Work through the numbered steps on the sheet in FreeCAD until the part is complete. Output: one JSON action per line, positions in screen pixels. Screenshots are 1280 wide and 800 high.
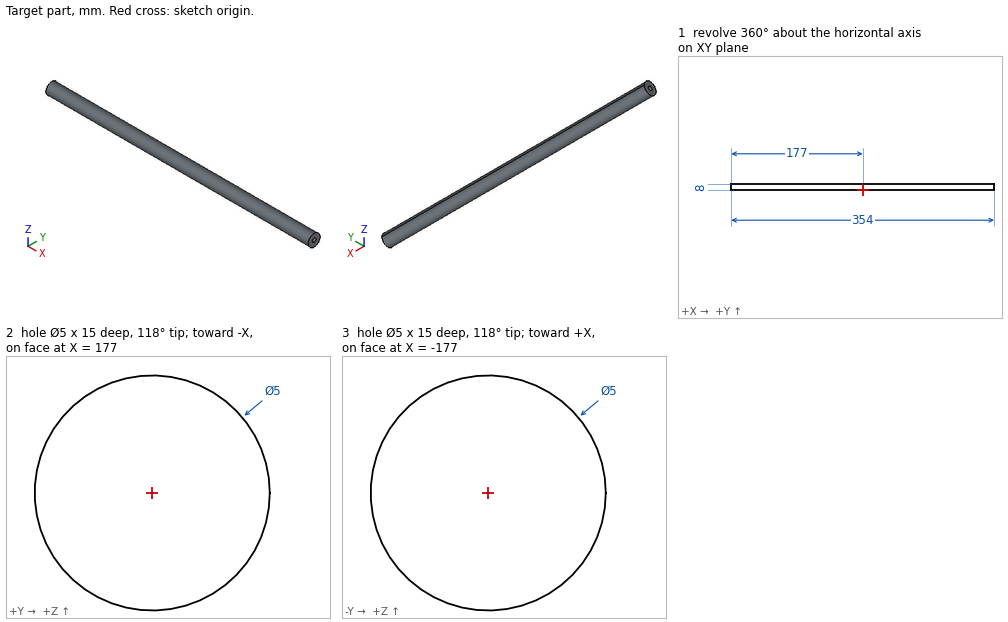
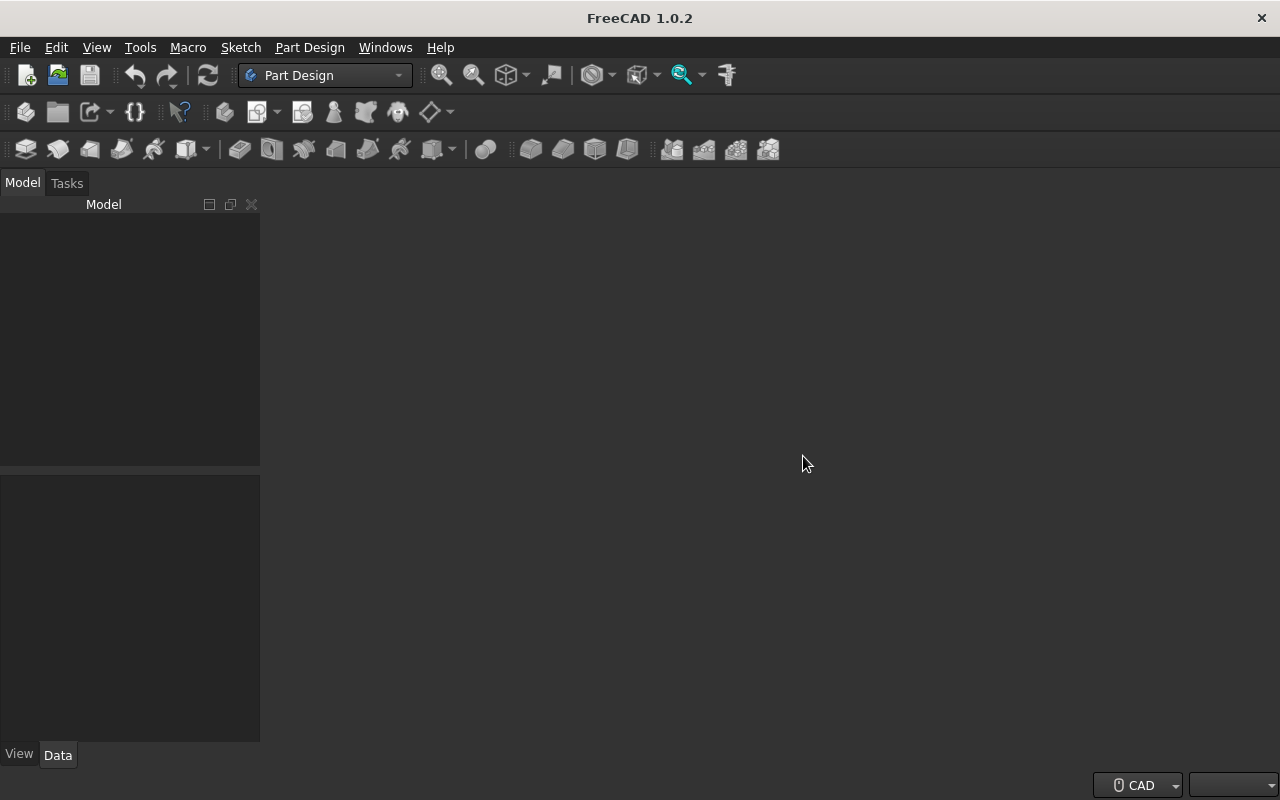
{"action": "left_click", "coordinate": [26, 76]}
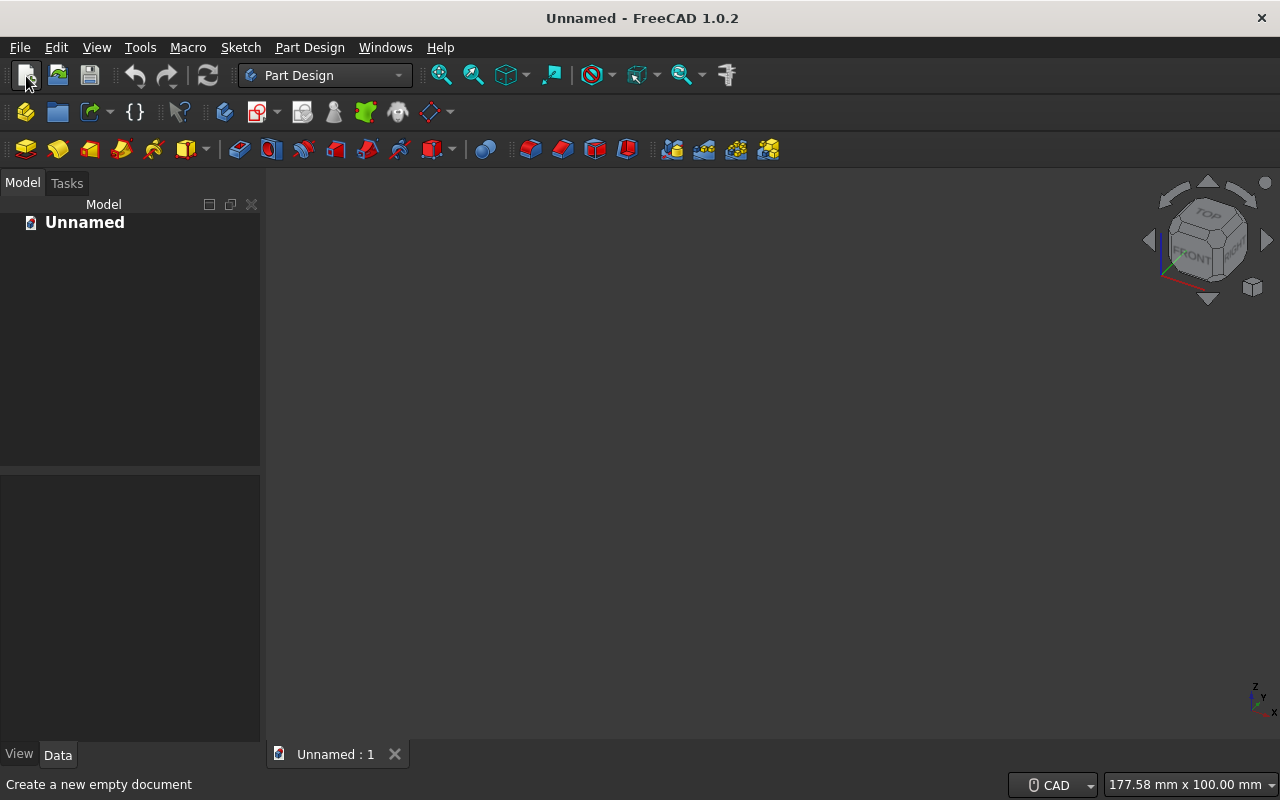
{"action": "left_click", "coordinate": [258, 112]}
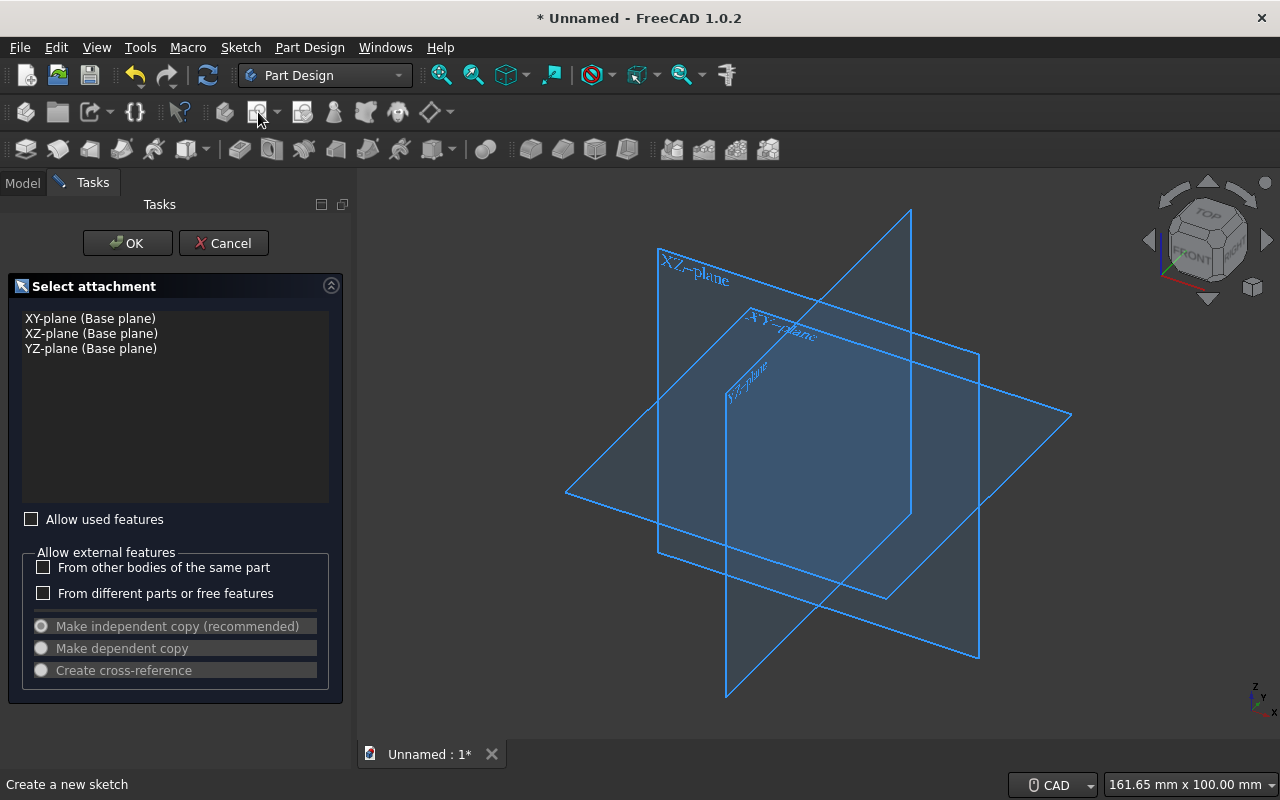
{"action": "left_click", "coordinate": [82, 318]}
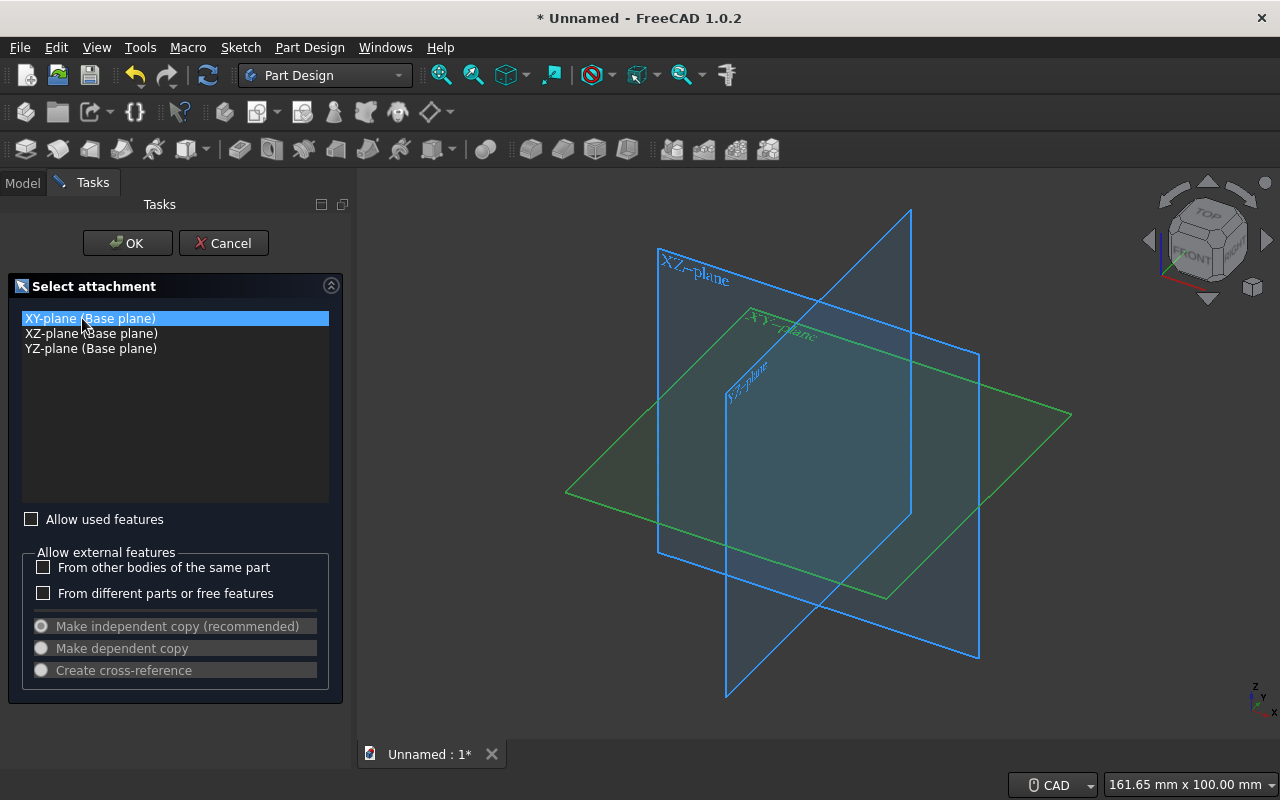
{"action": "left_click", "coordinate": [128, 243]}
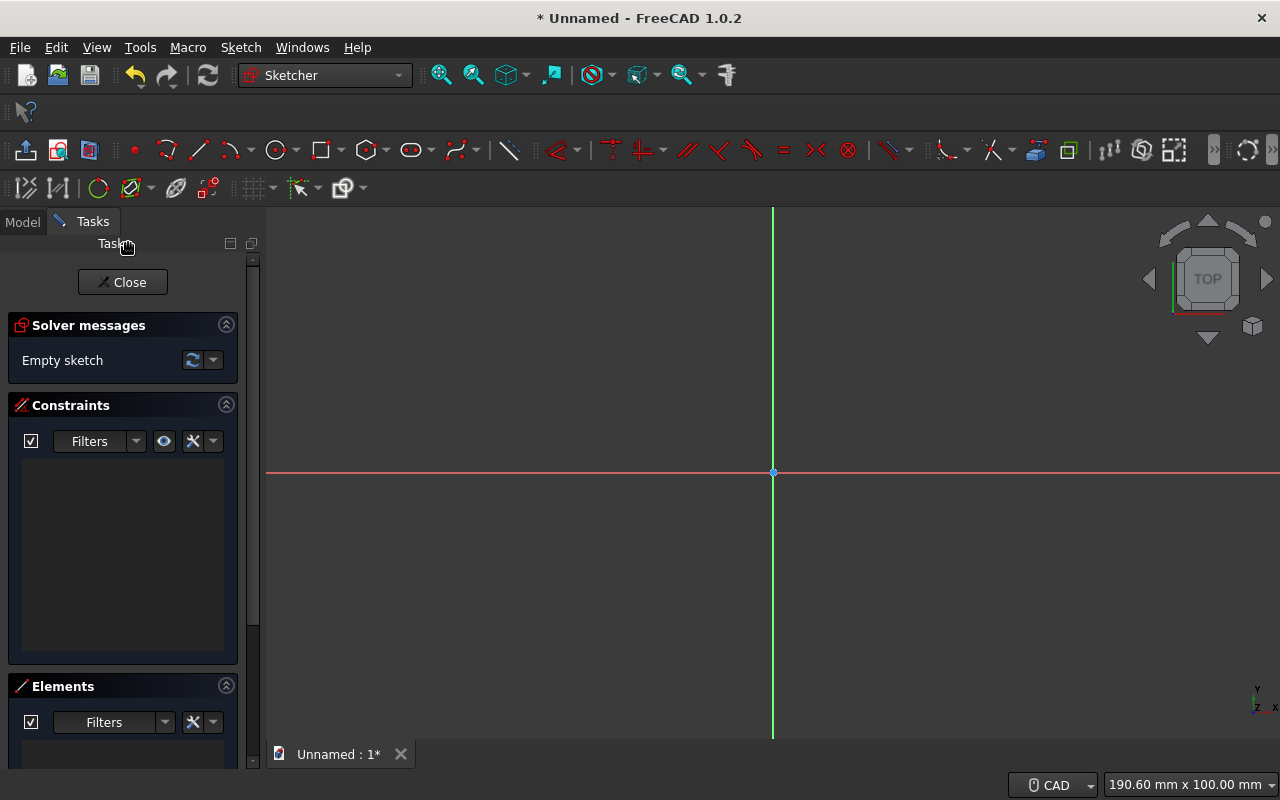
{"action": "scroll", "coordinate": [675, 482], "scroll_direction": "down", "scroll_amount": 6}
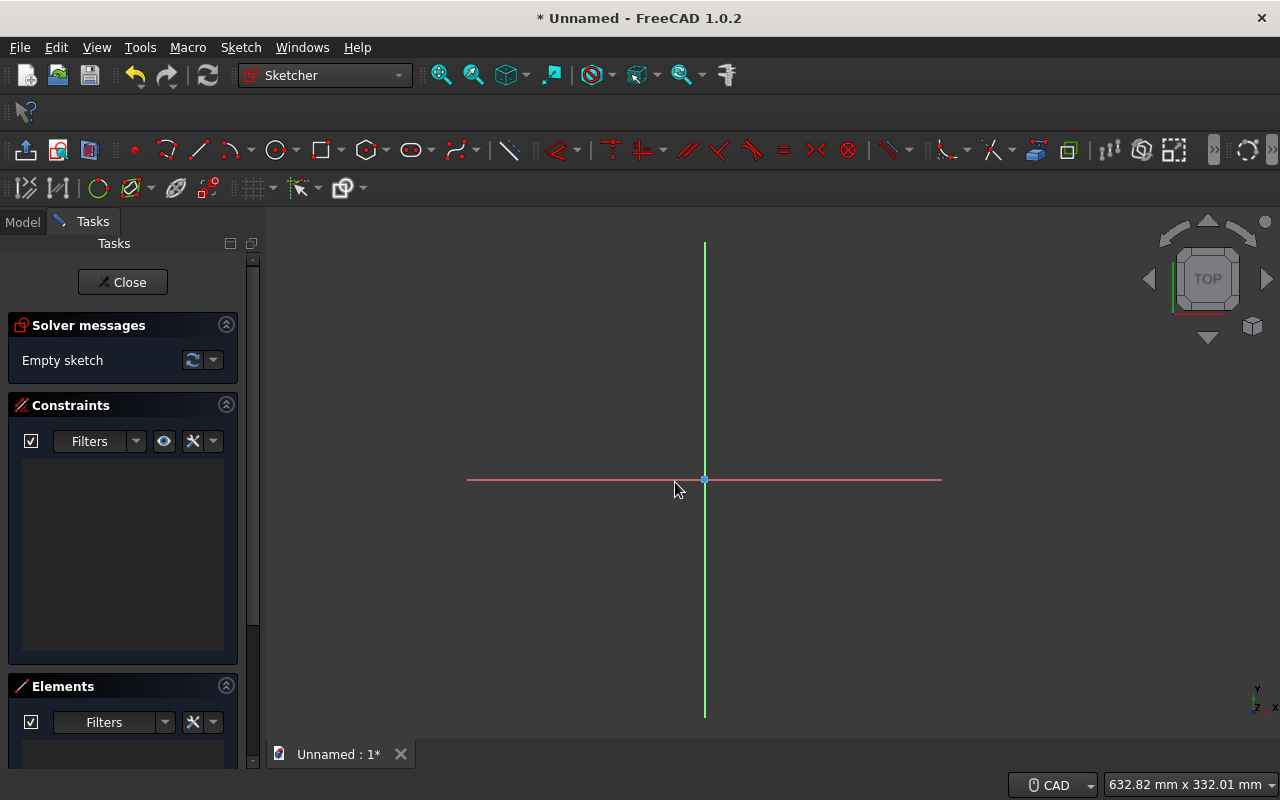
{"action": "key", "text": "g r"}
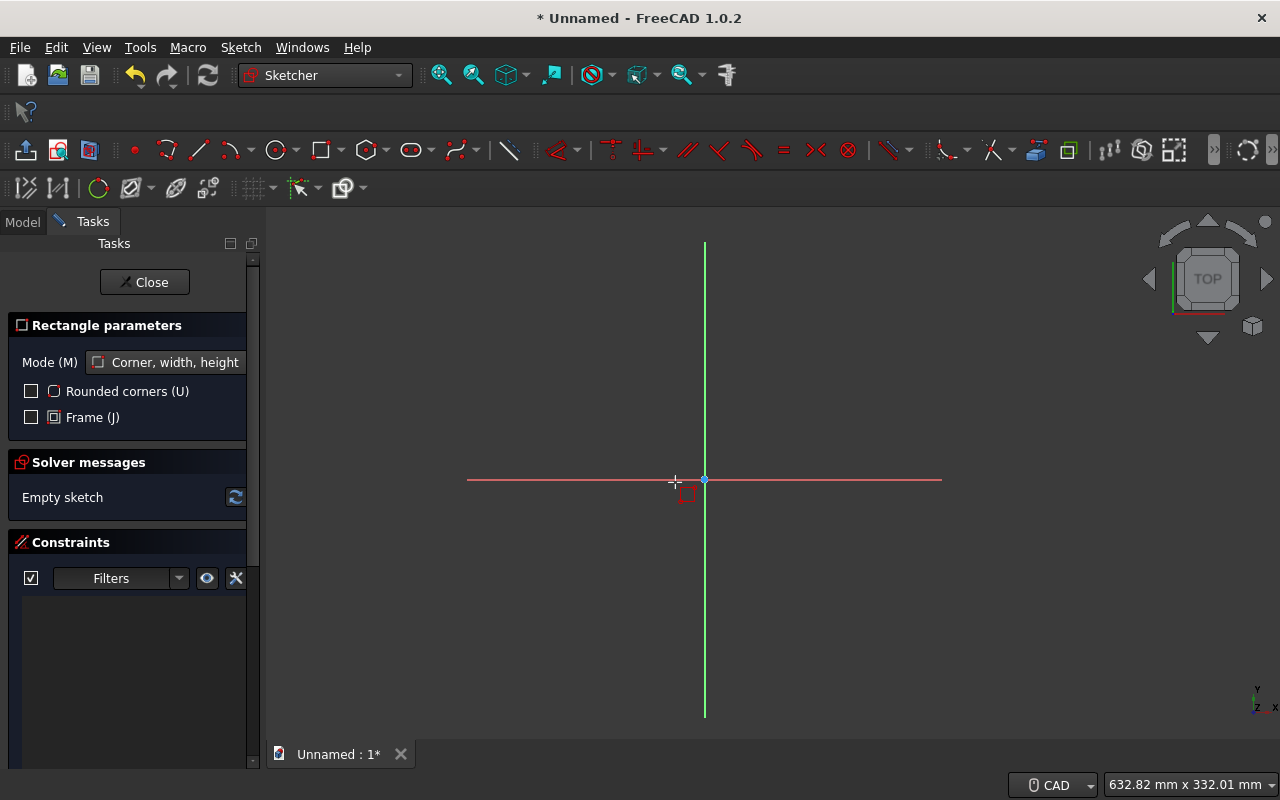
{"action": "scroll", "coordinate": [421, 467], "scroll_direction": "up", "scroll_amount": 2}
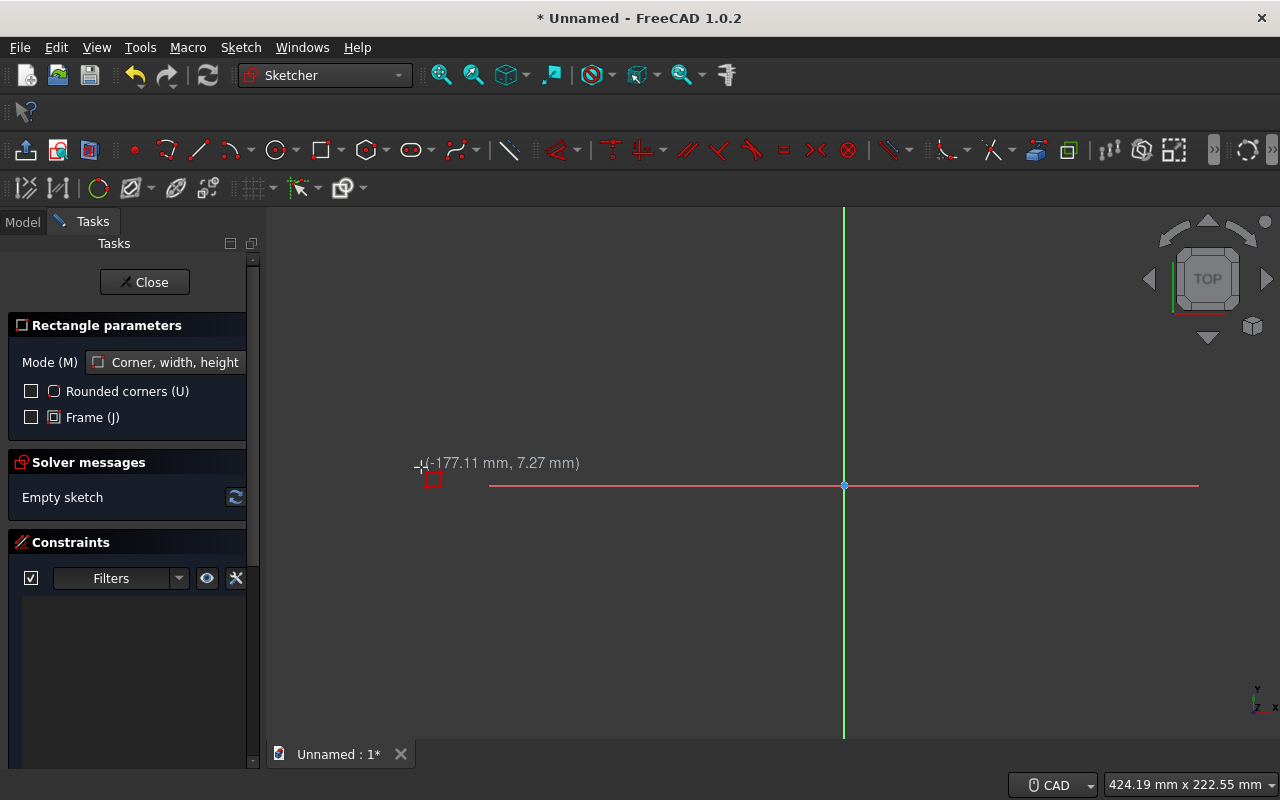
{"action": "left_click", "coordinate": [421, 467]}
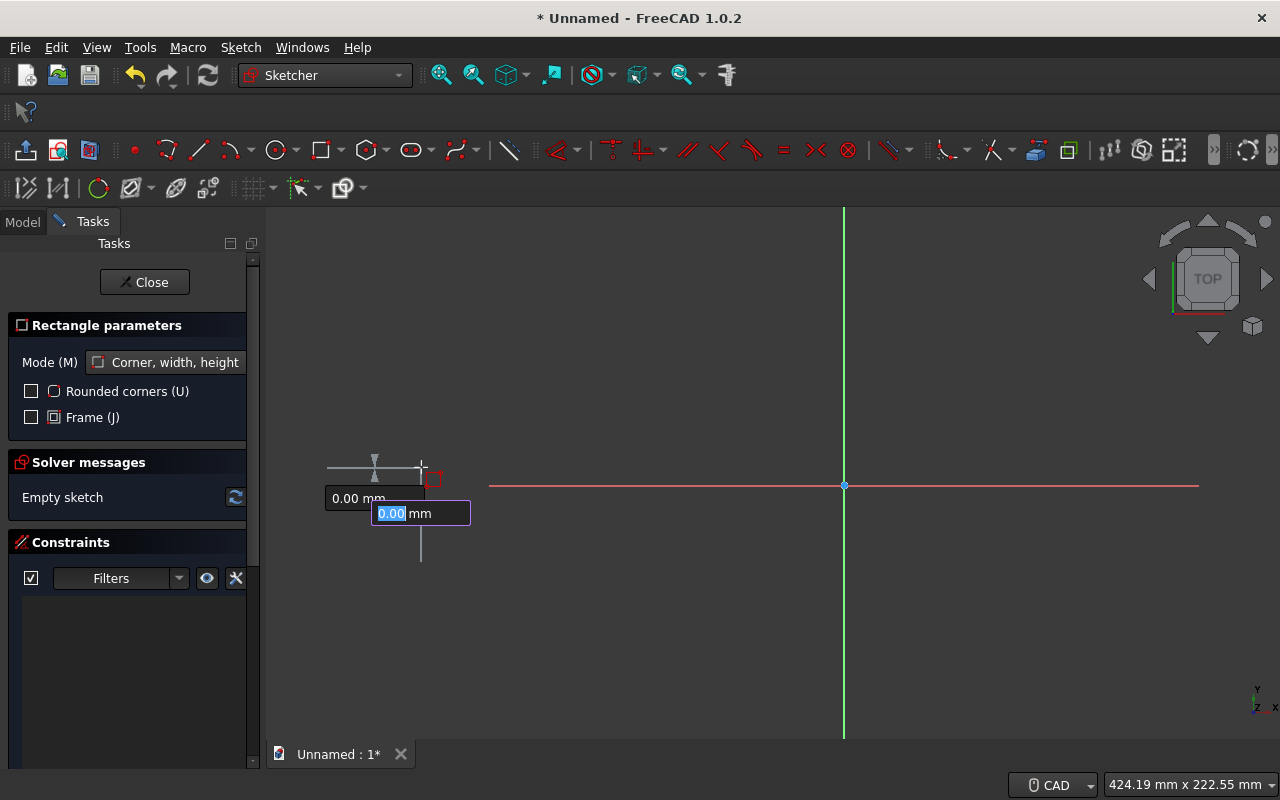
{"action": "scroll", "coordinate": [420, 467], "scroll_direction": "down", "scroll_amount": 2}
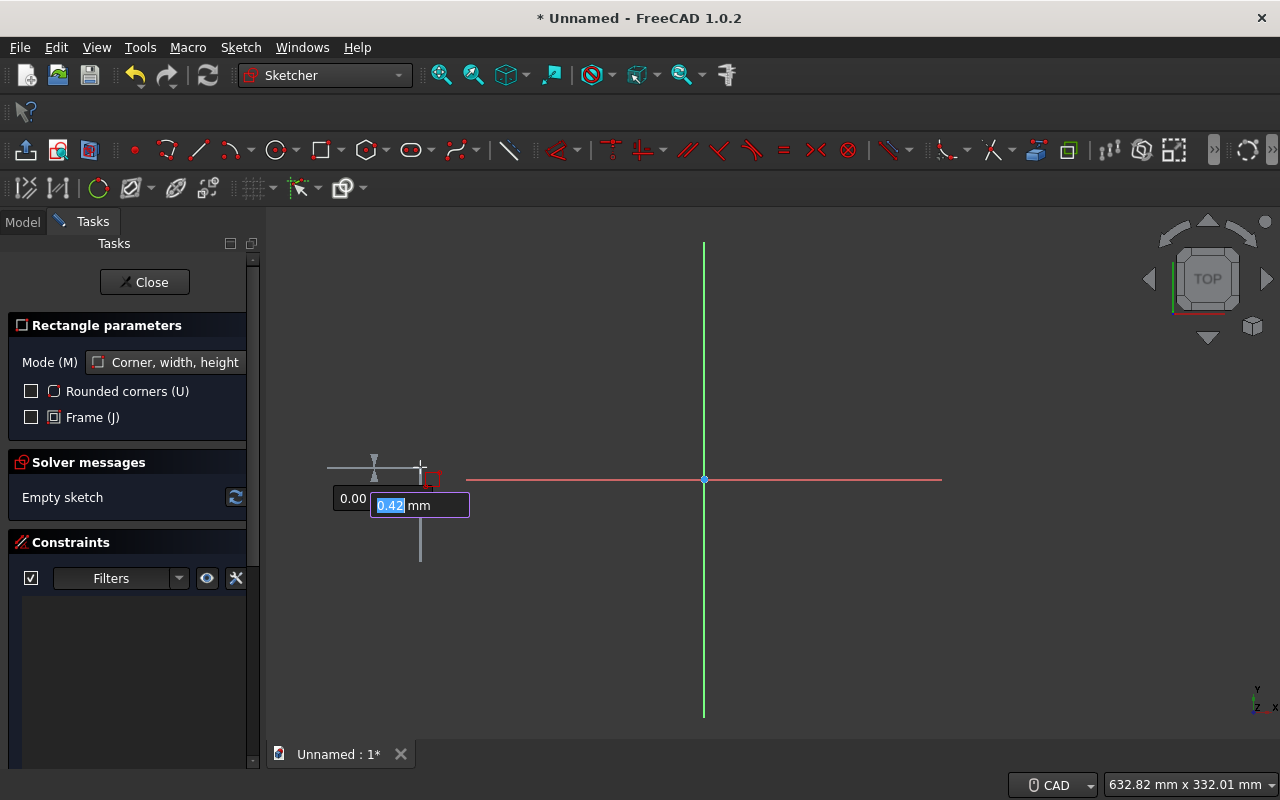
{"action": "left_click", "coordinate": [988, 480]}
{"action": "key", "text": "Escape"}